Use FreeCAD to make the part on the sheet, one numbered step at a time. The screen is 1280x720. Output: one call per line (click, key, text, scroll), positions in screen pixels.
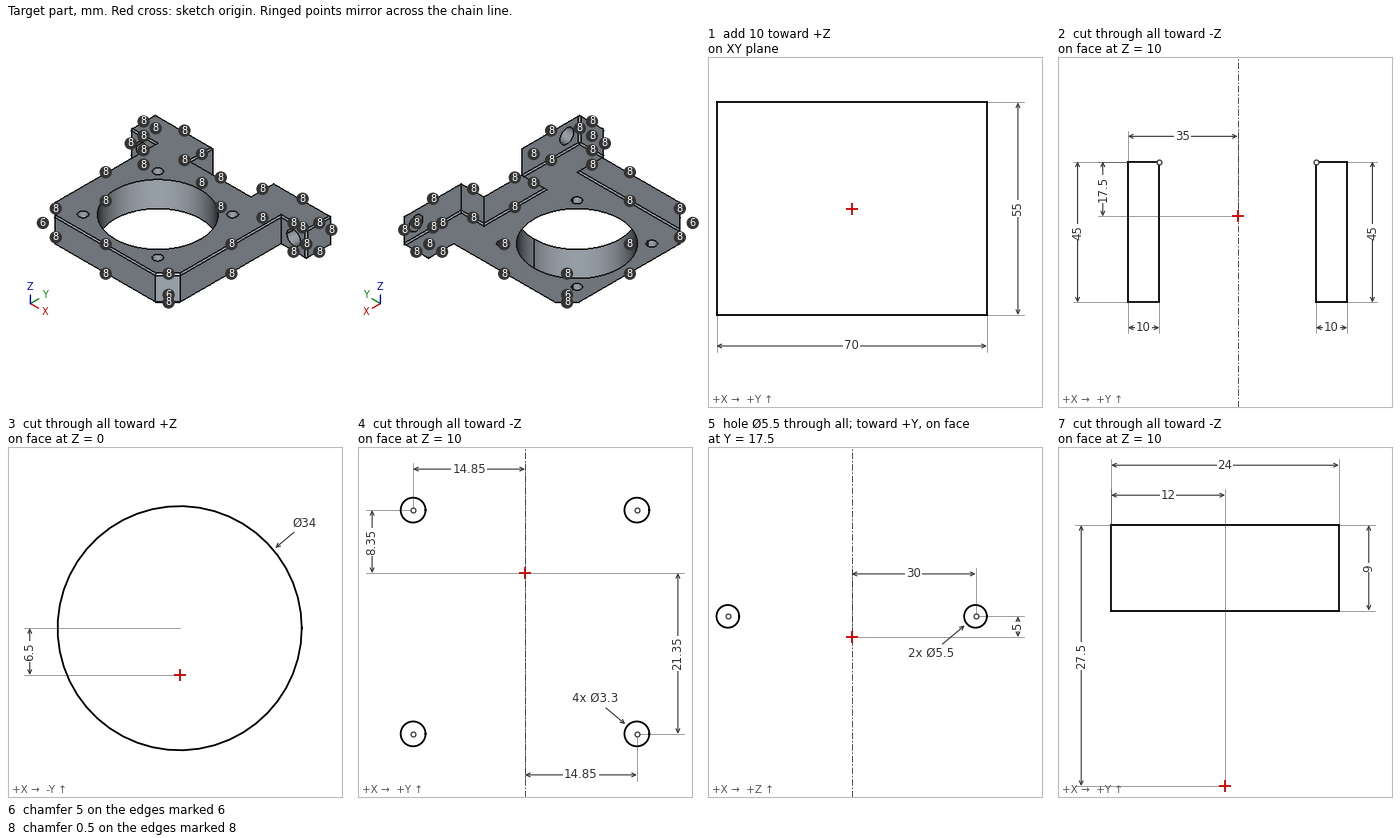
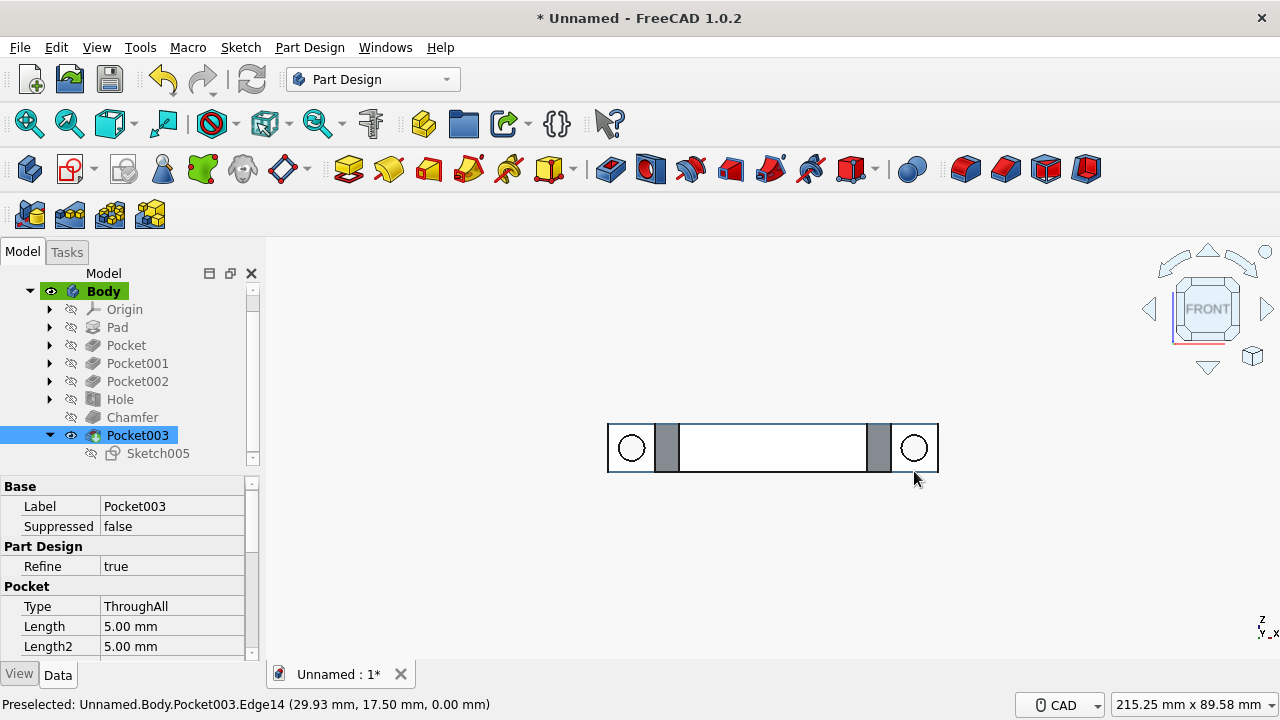
click(773, 471, ctrl)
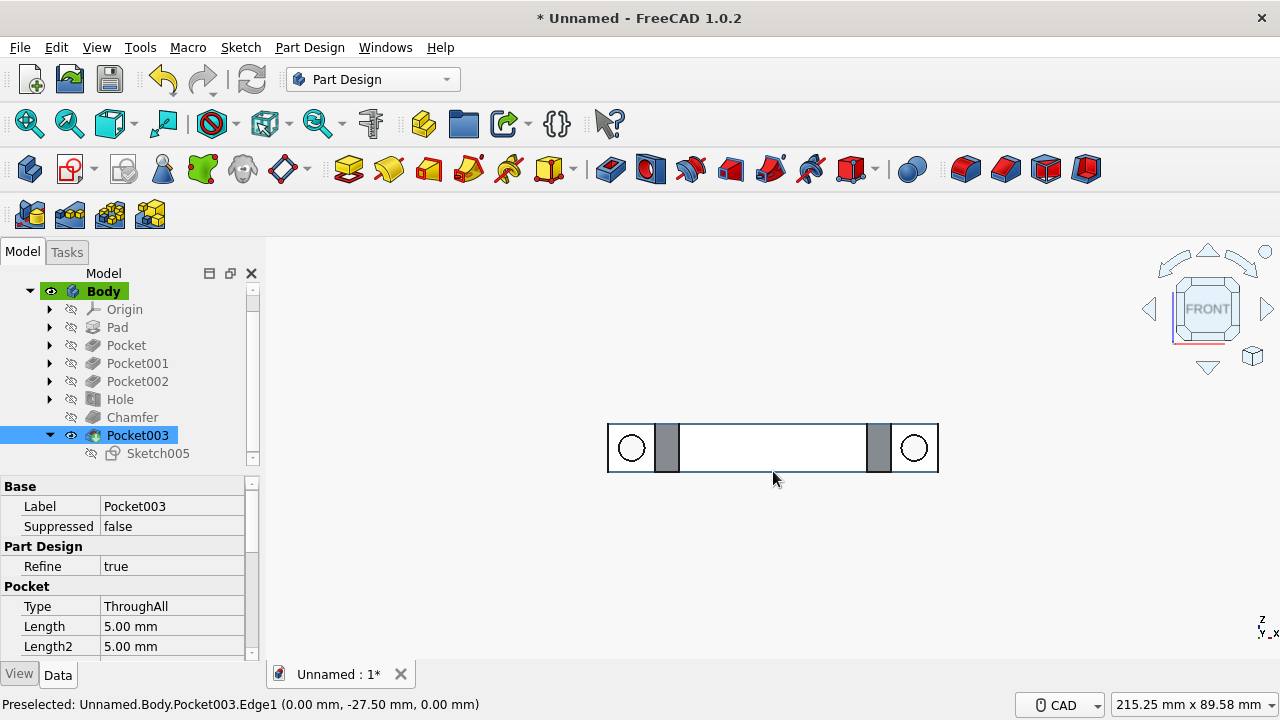
click(879, 471, ctrl)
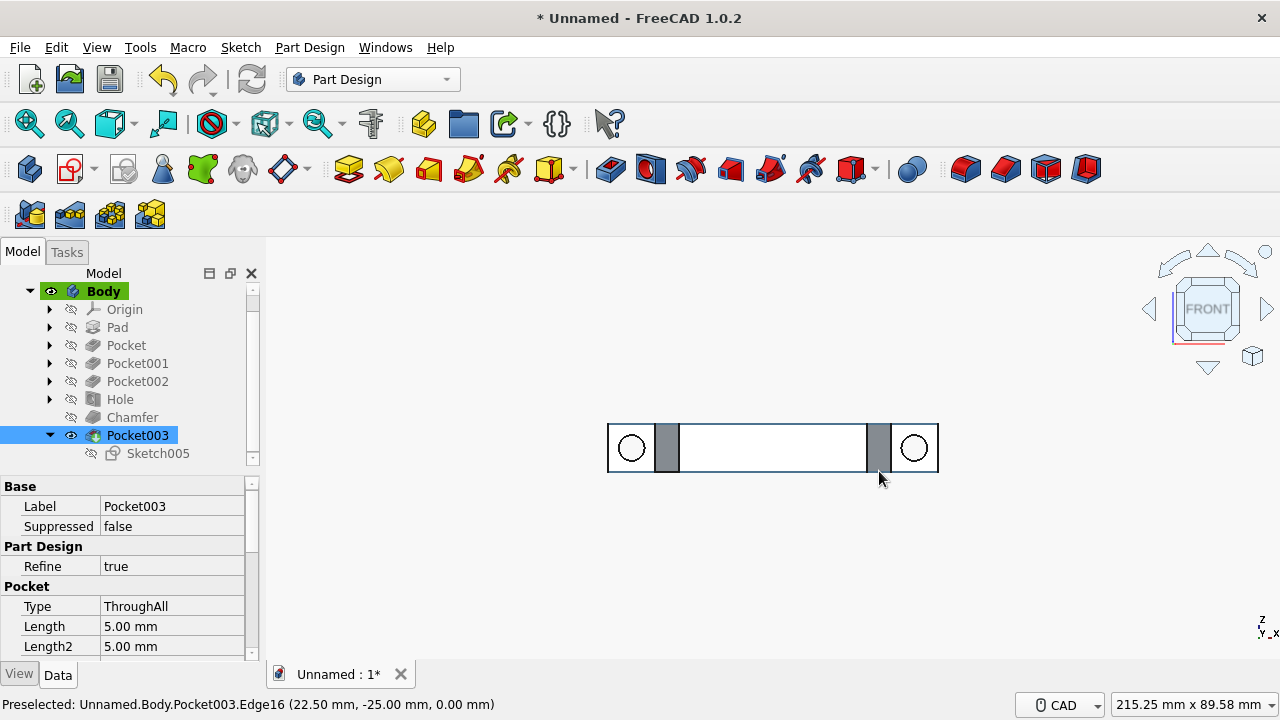
click(667, 471, ctrl)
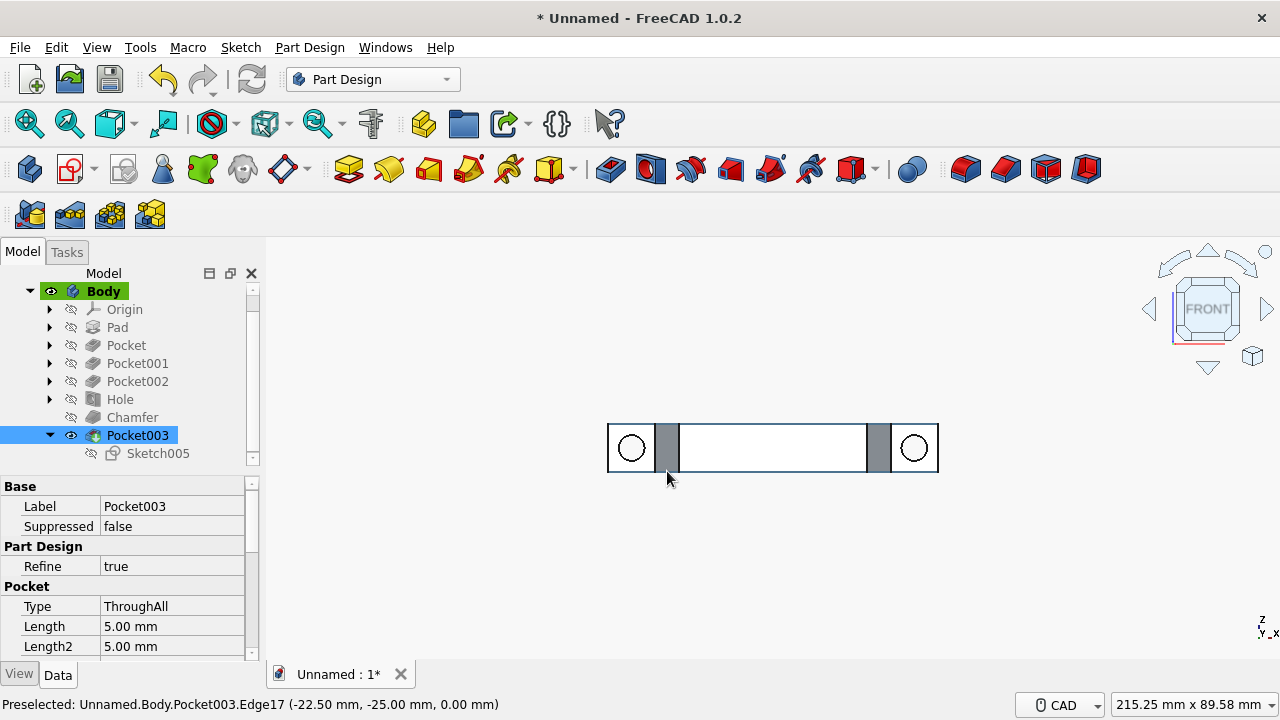
key(3)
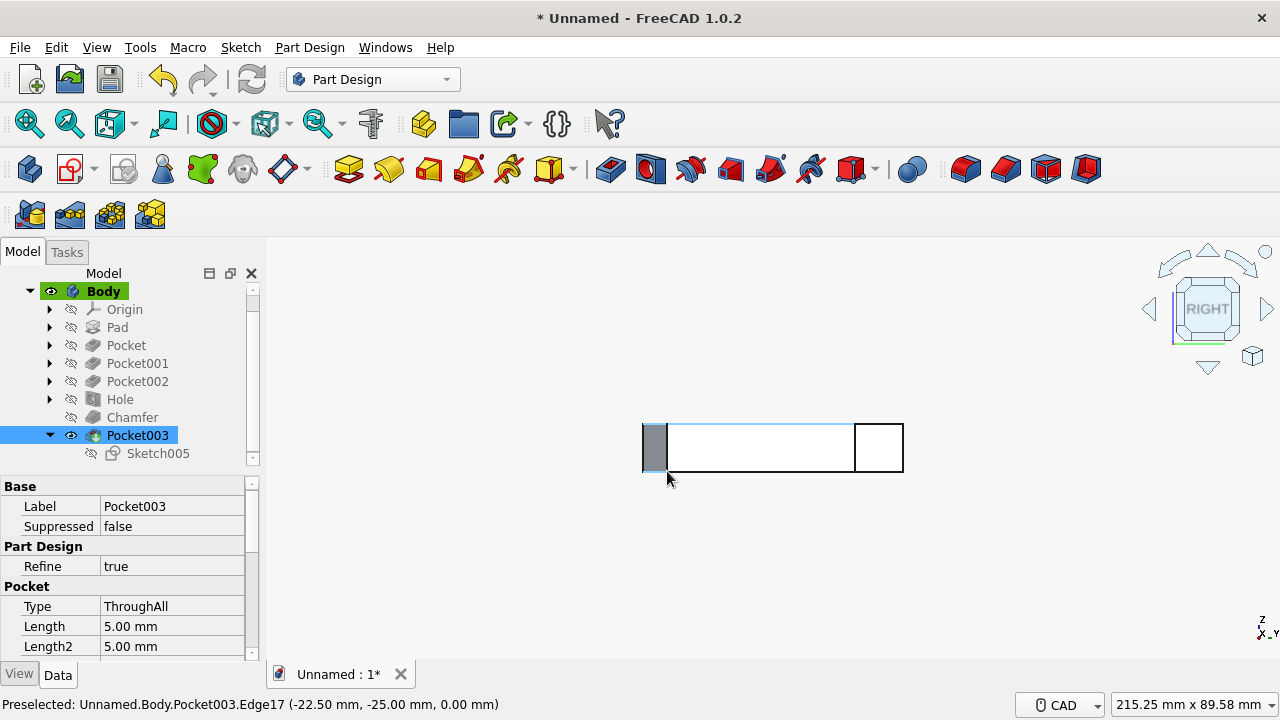
key(v)
key(f)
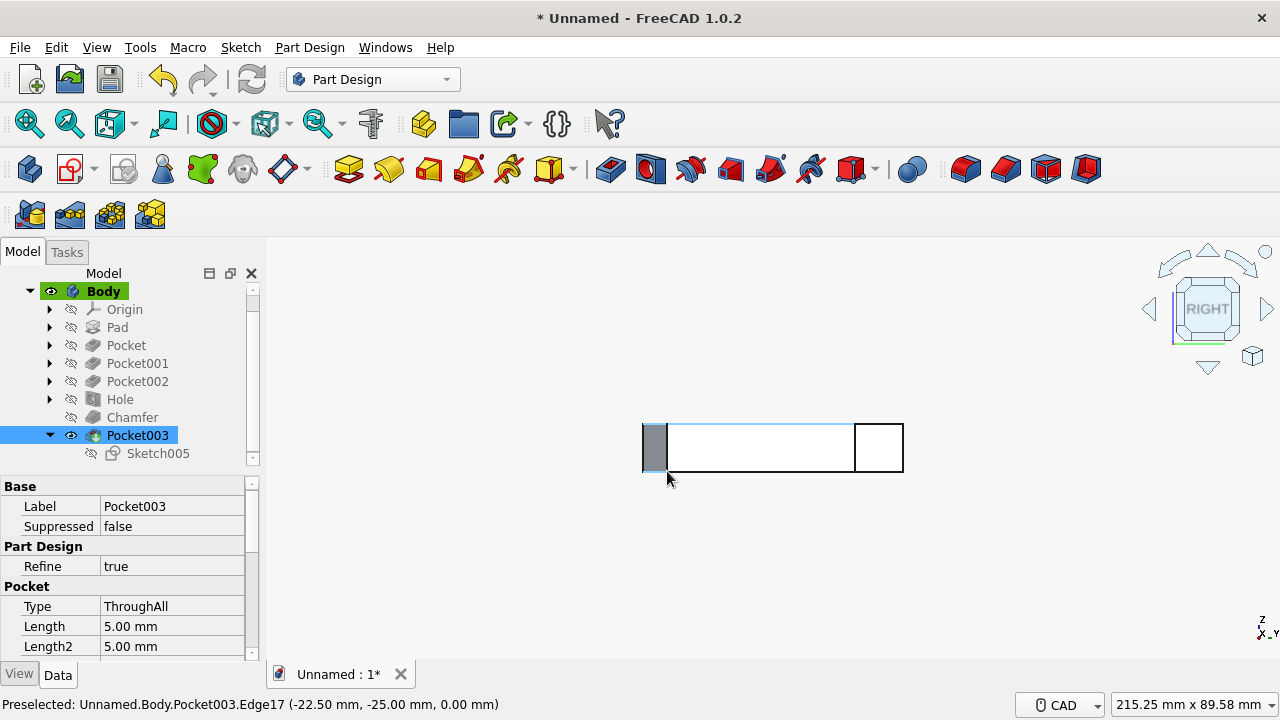
click(761, 471, ctrl)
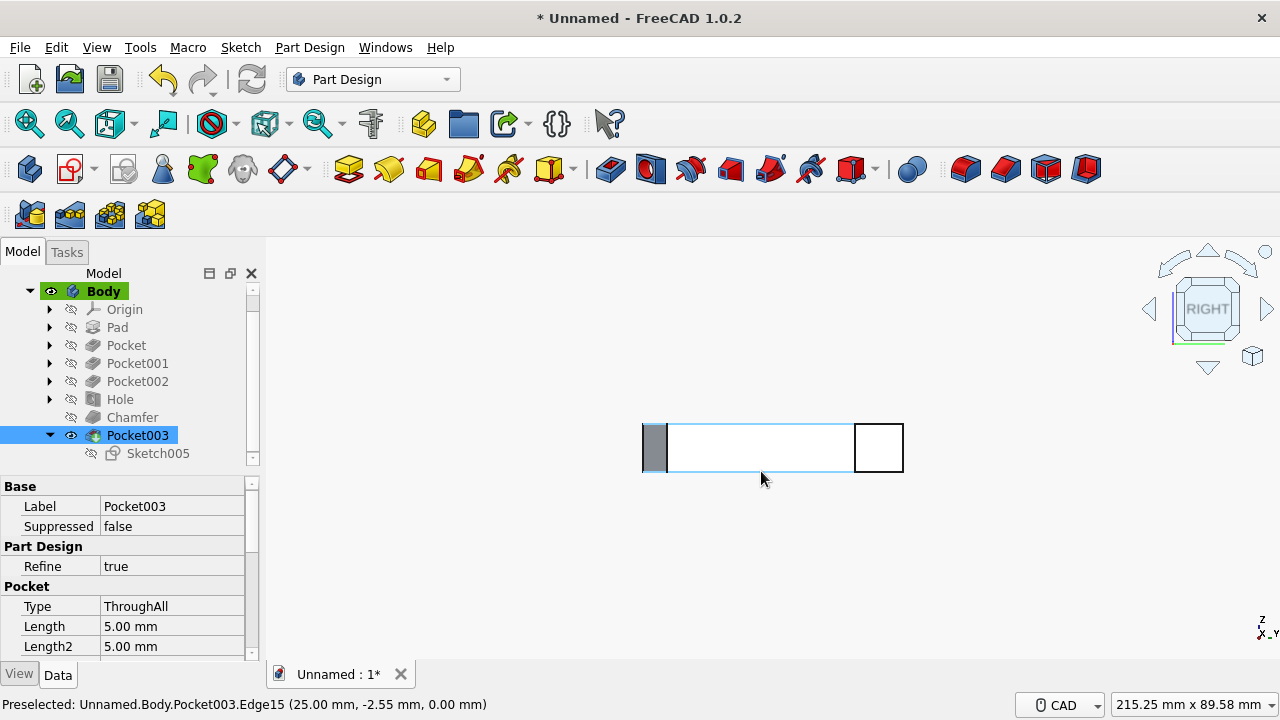
key(5)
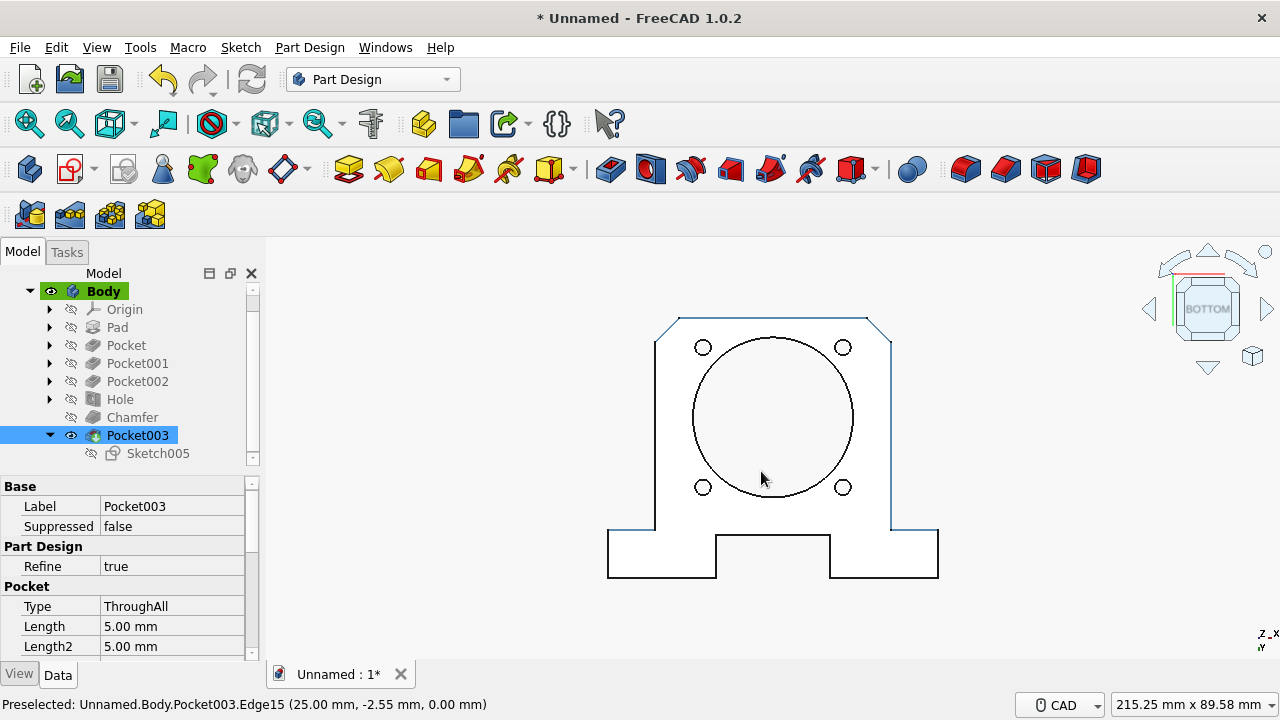
click(884, 577, ctrl)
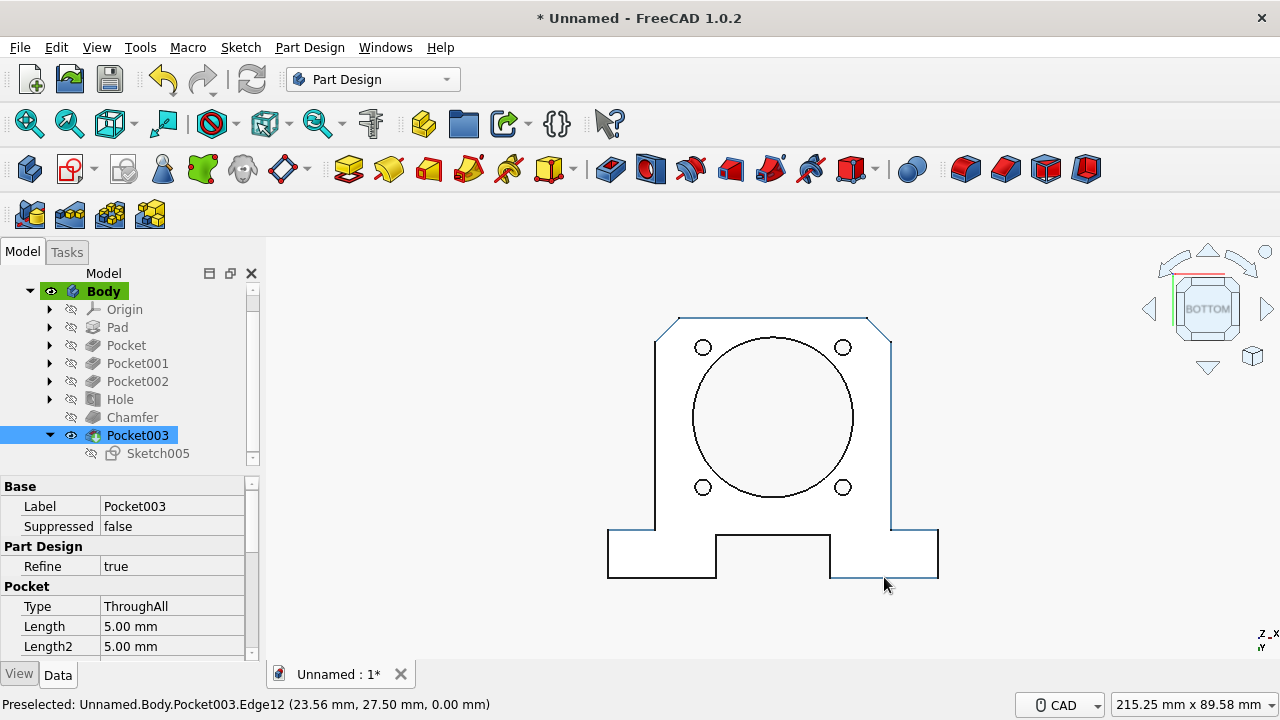
click(655, 435, ctrl)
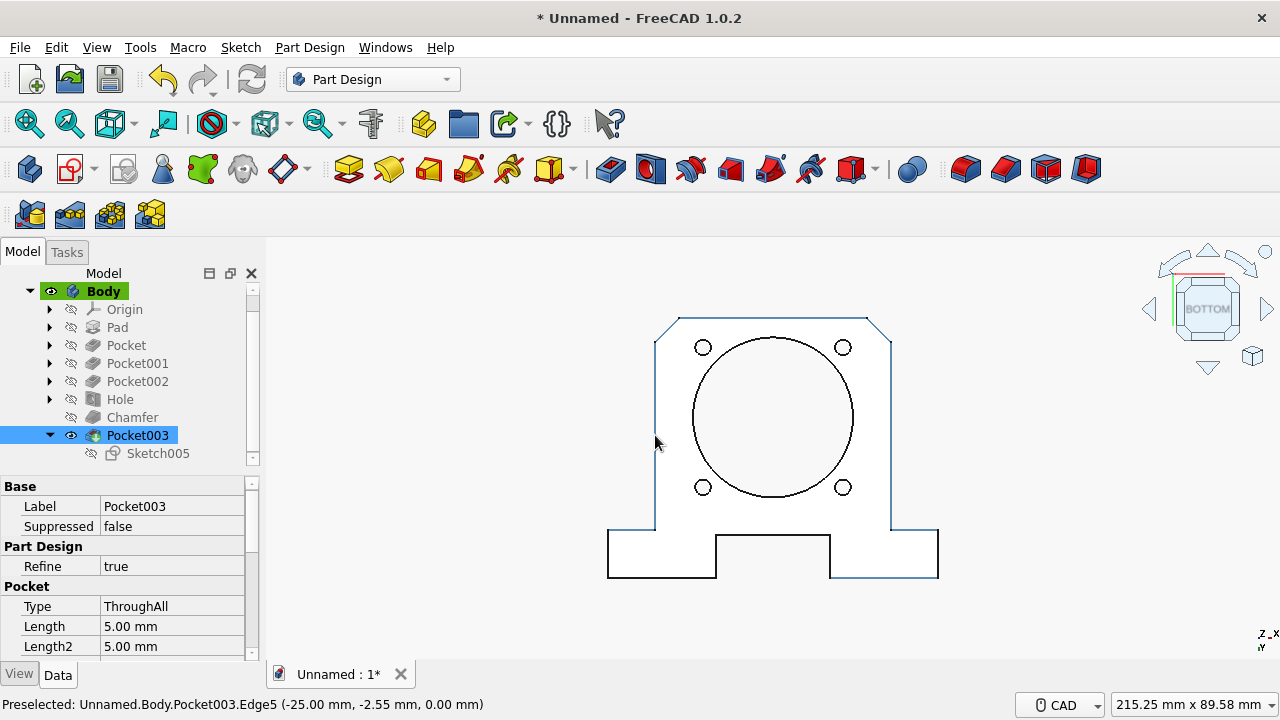
click(662, 577, ctrl)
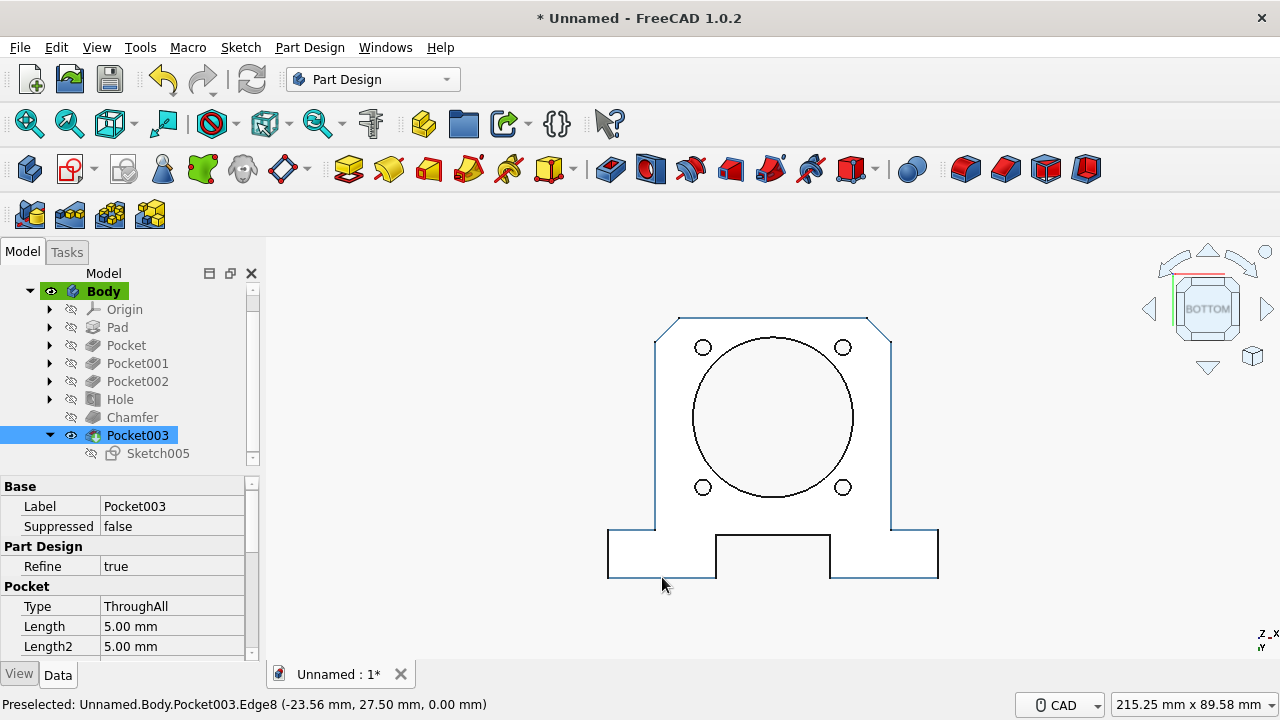
click(716, 555, ctrl)